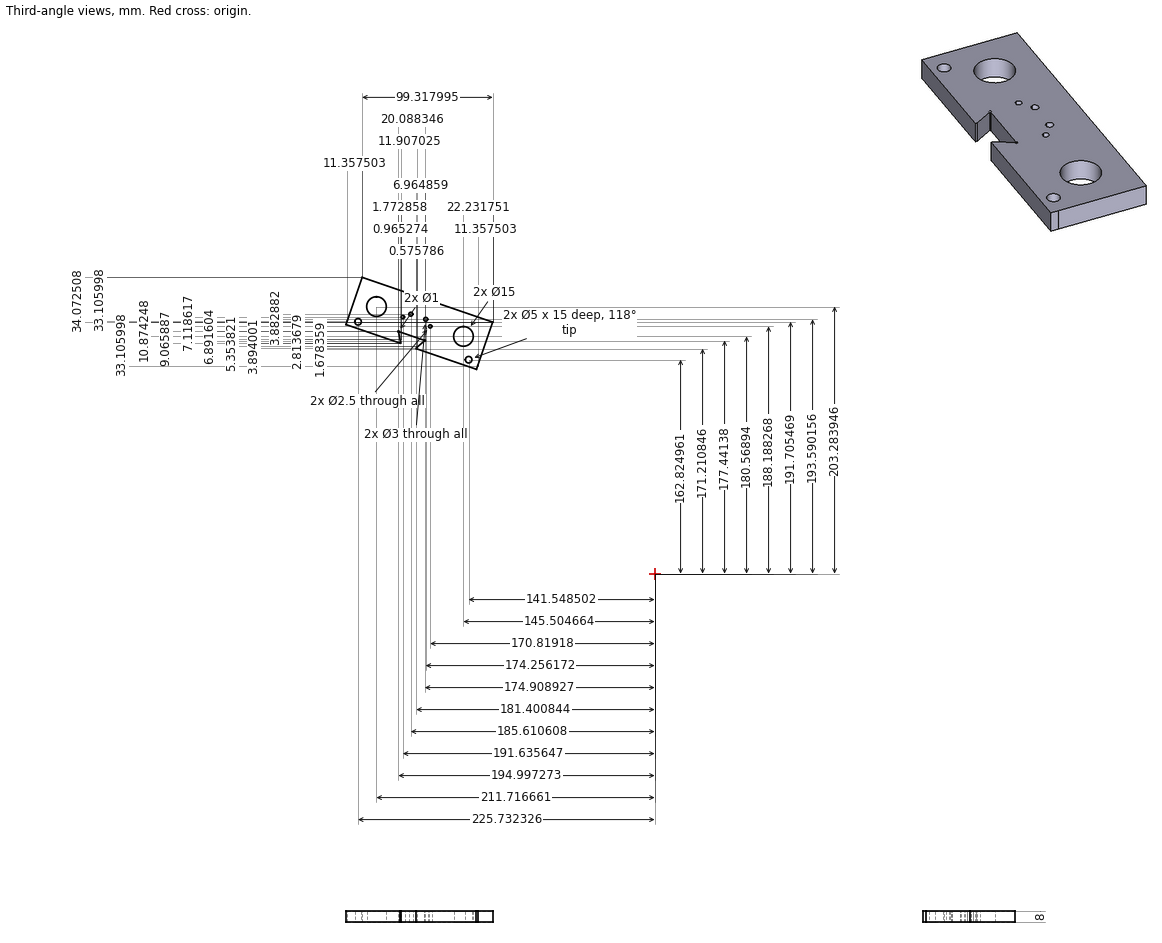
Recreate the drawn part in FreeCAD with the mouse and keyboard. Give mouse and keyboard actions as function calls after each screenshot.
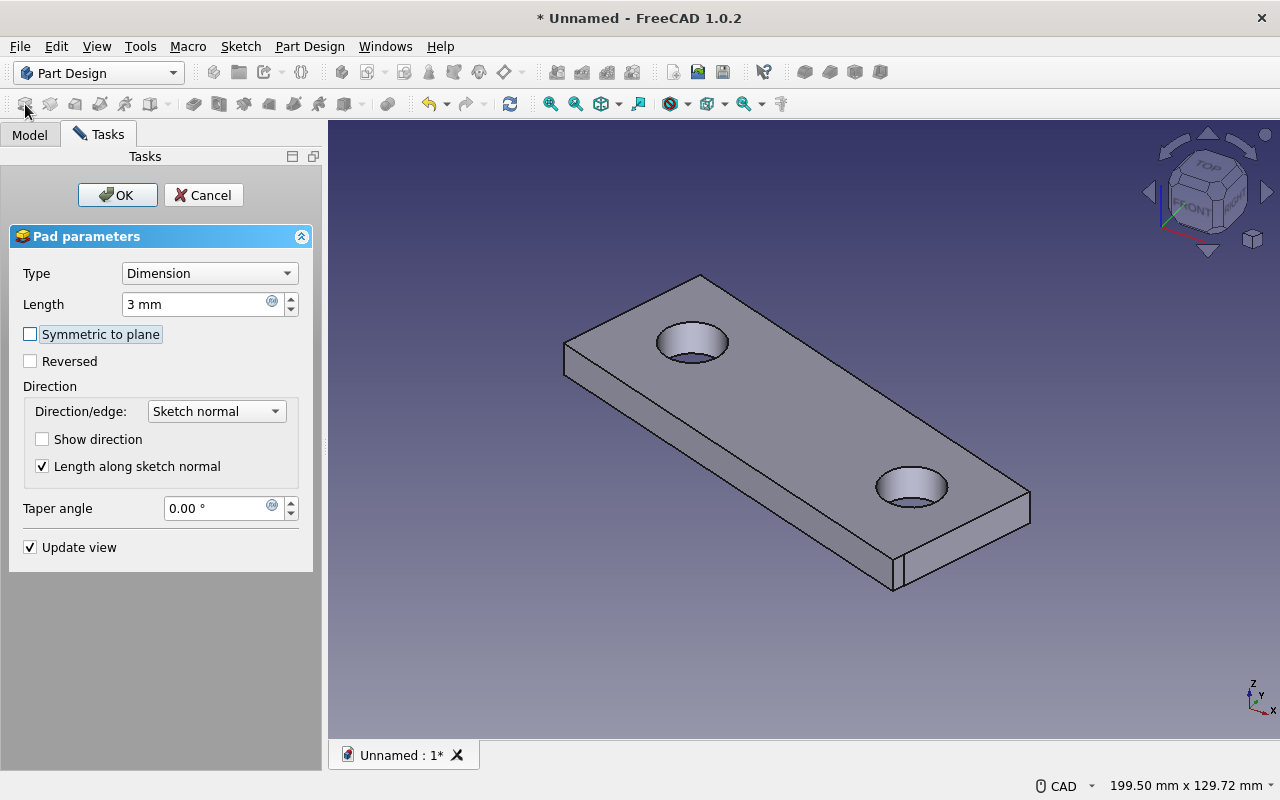
click(118, 195)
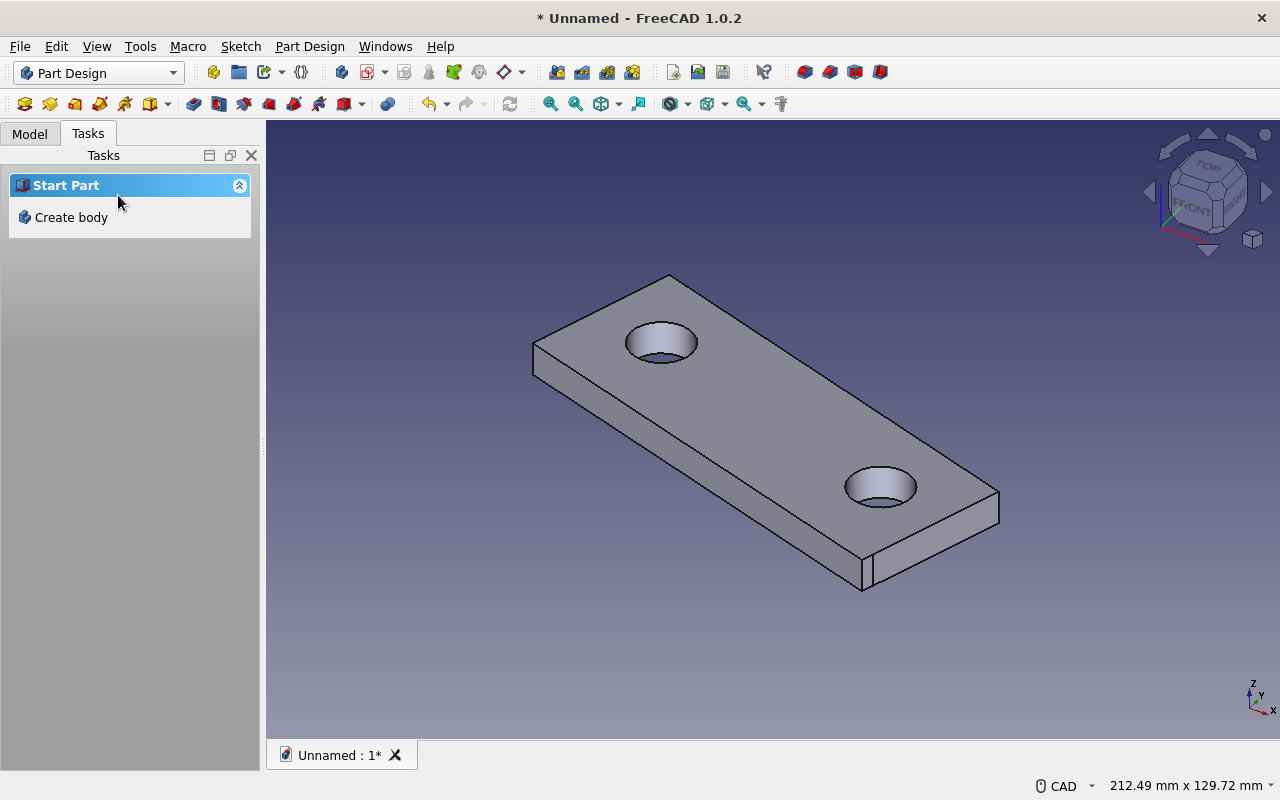
click(766, 416)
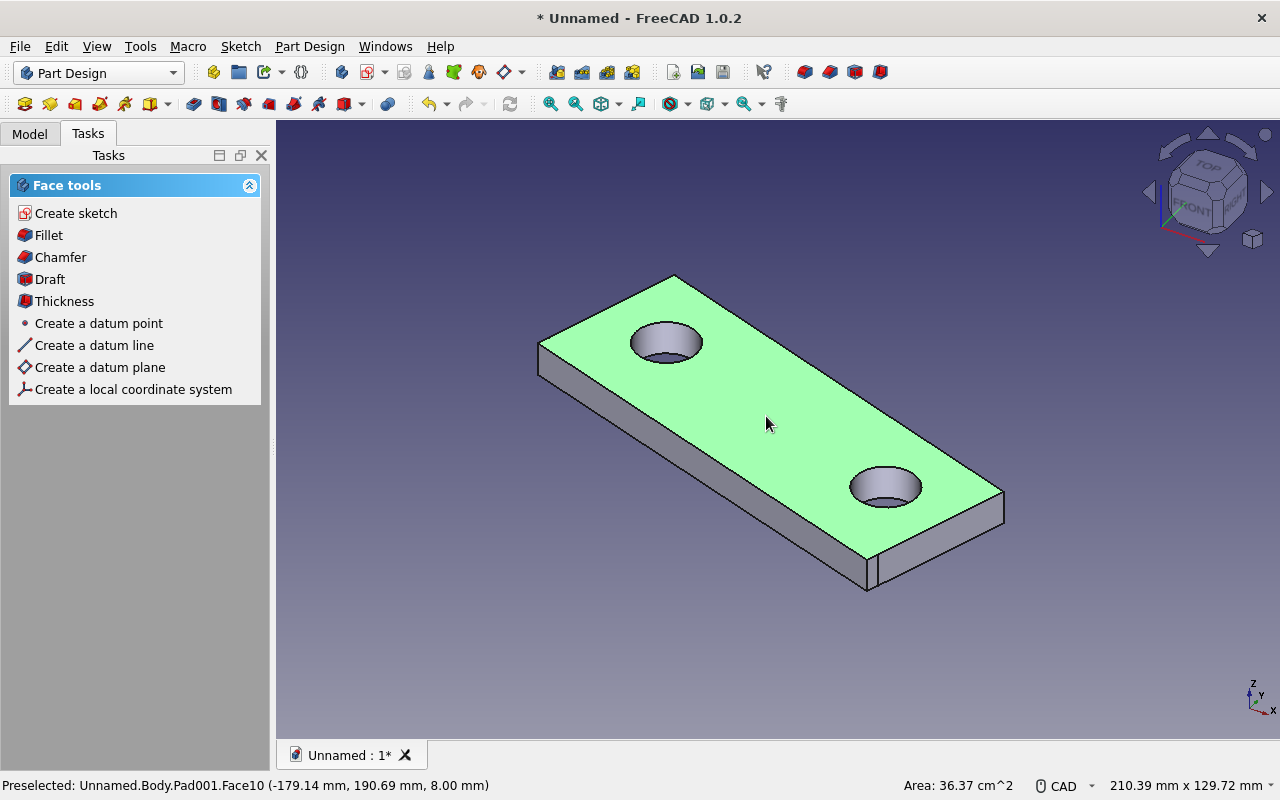
click(366, 72)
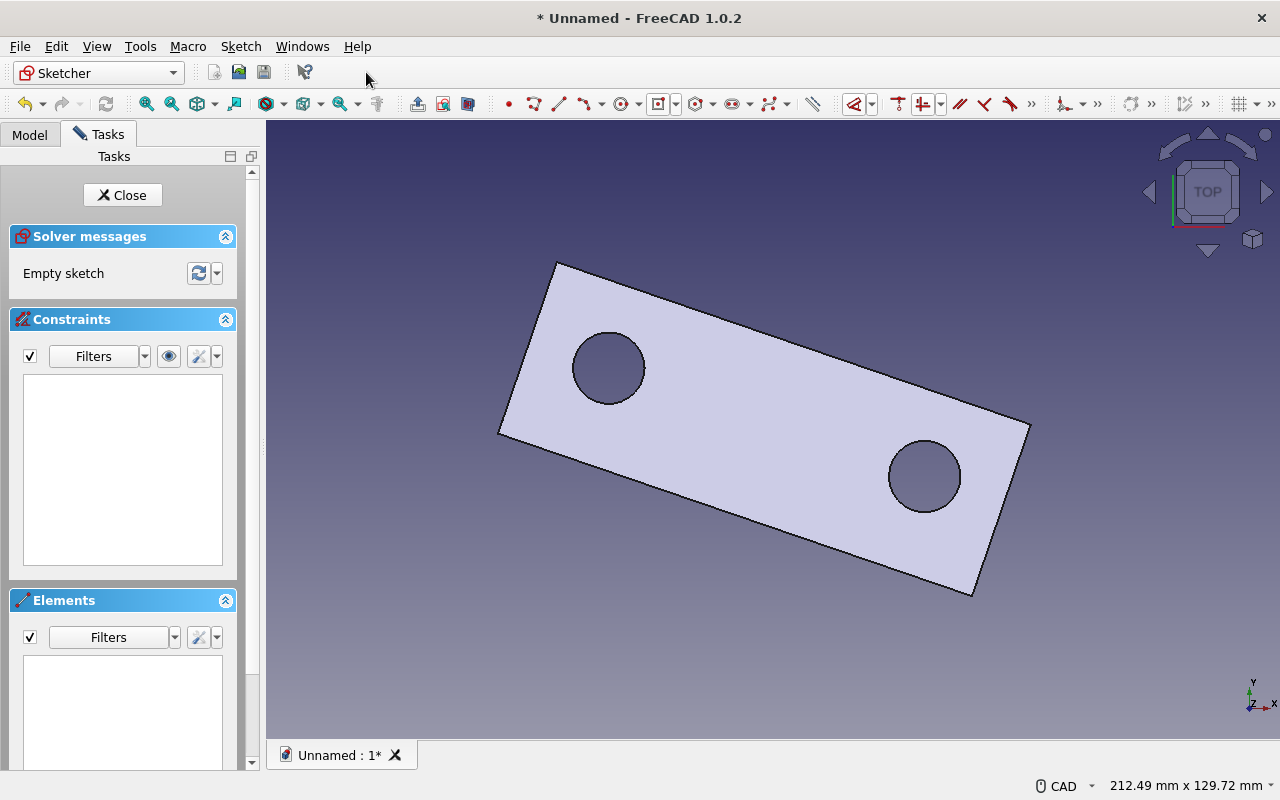
scroll(743, 501, up, 9)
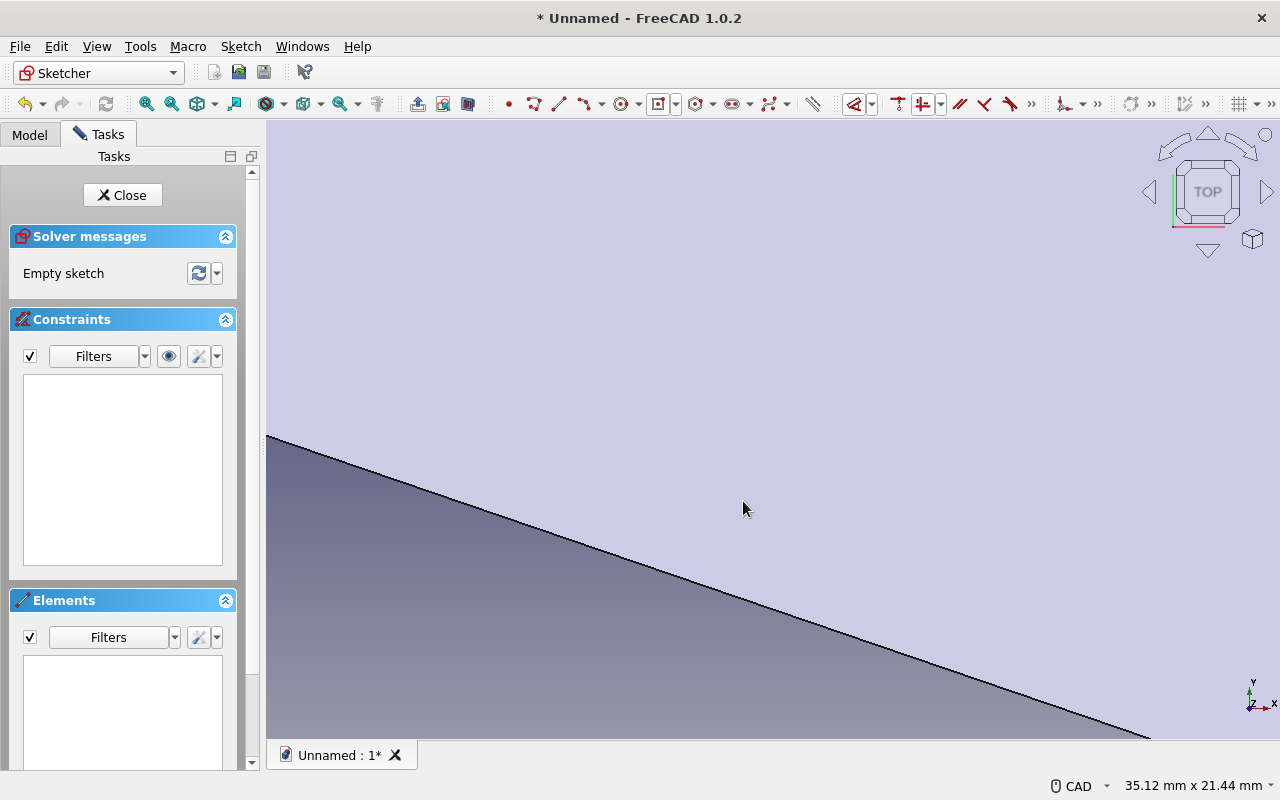
click(534, 104)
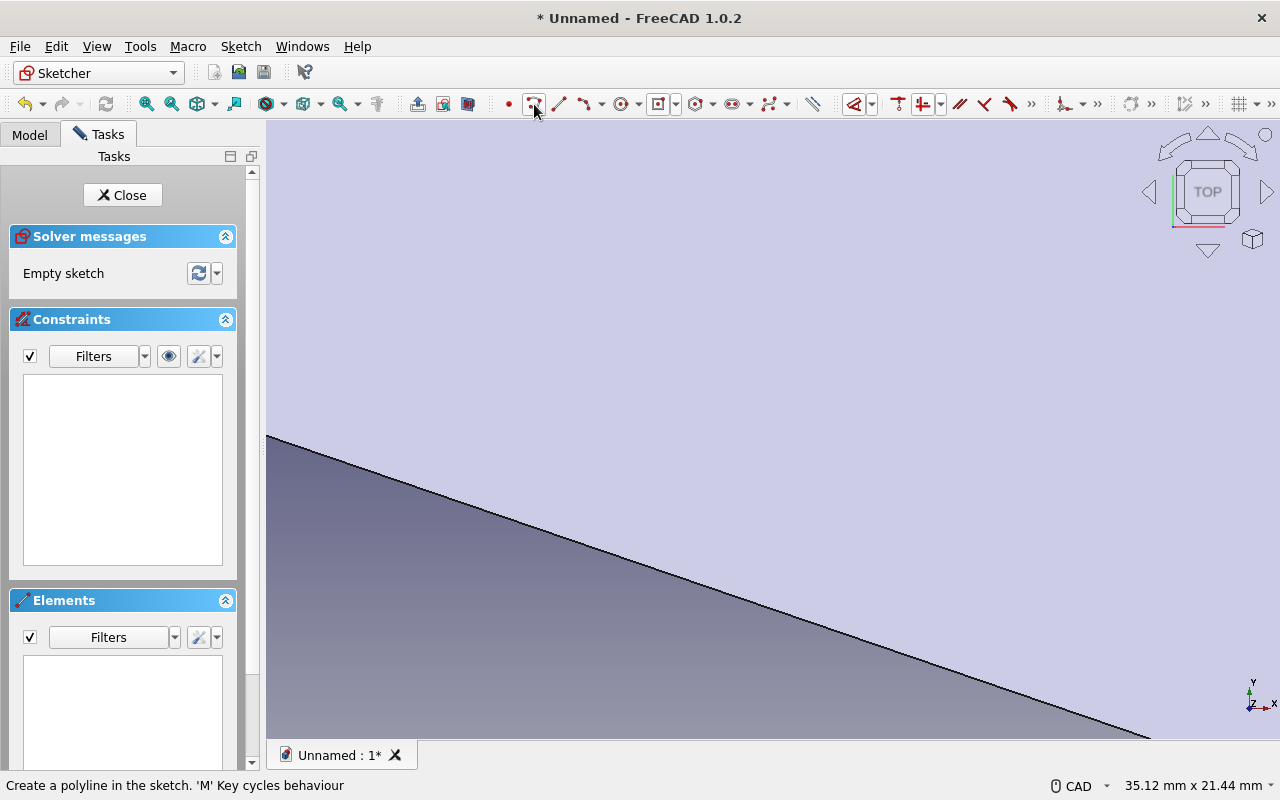
click(991, 440)
click(411, 241)
click(462, 503)
click(790, 615)
click(991, 441)
key(Escape)
key(Escape)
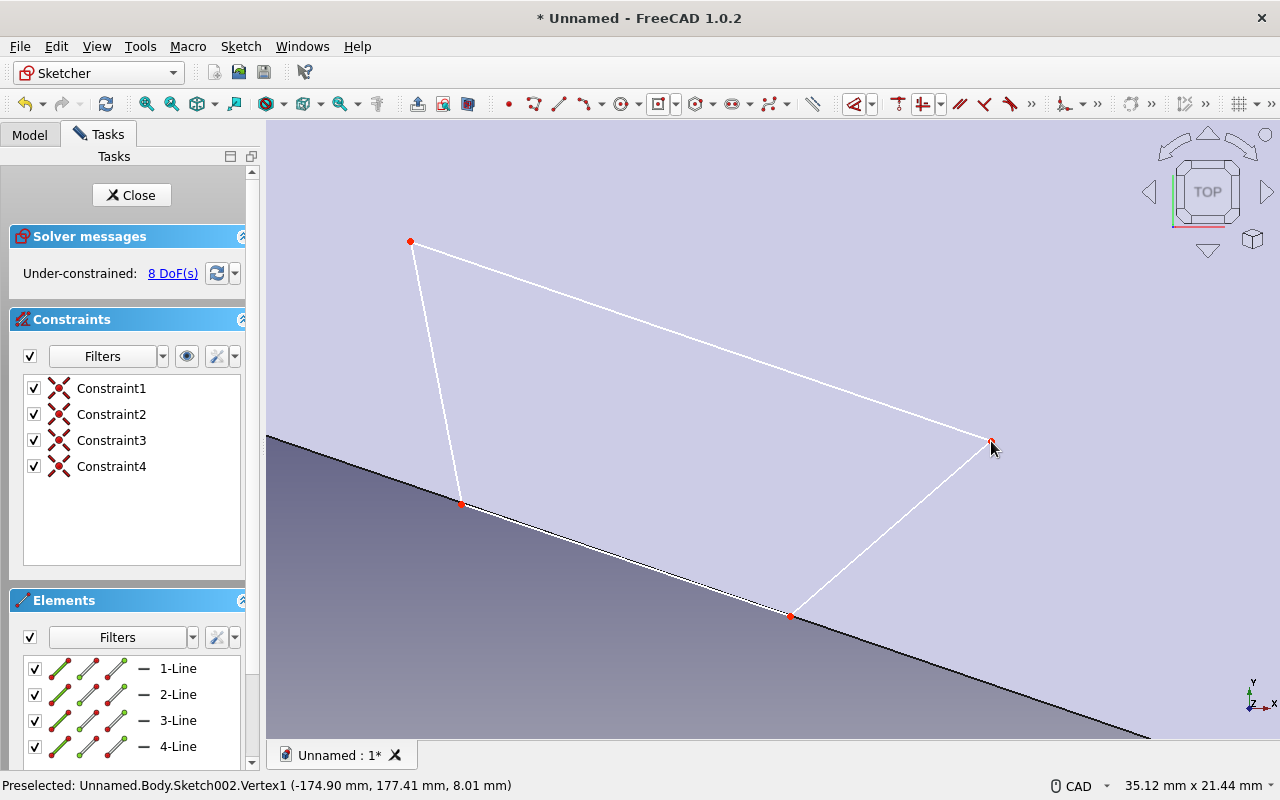
click(817, 381)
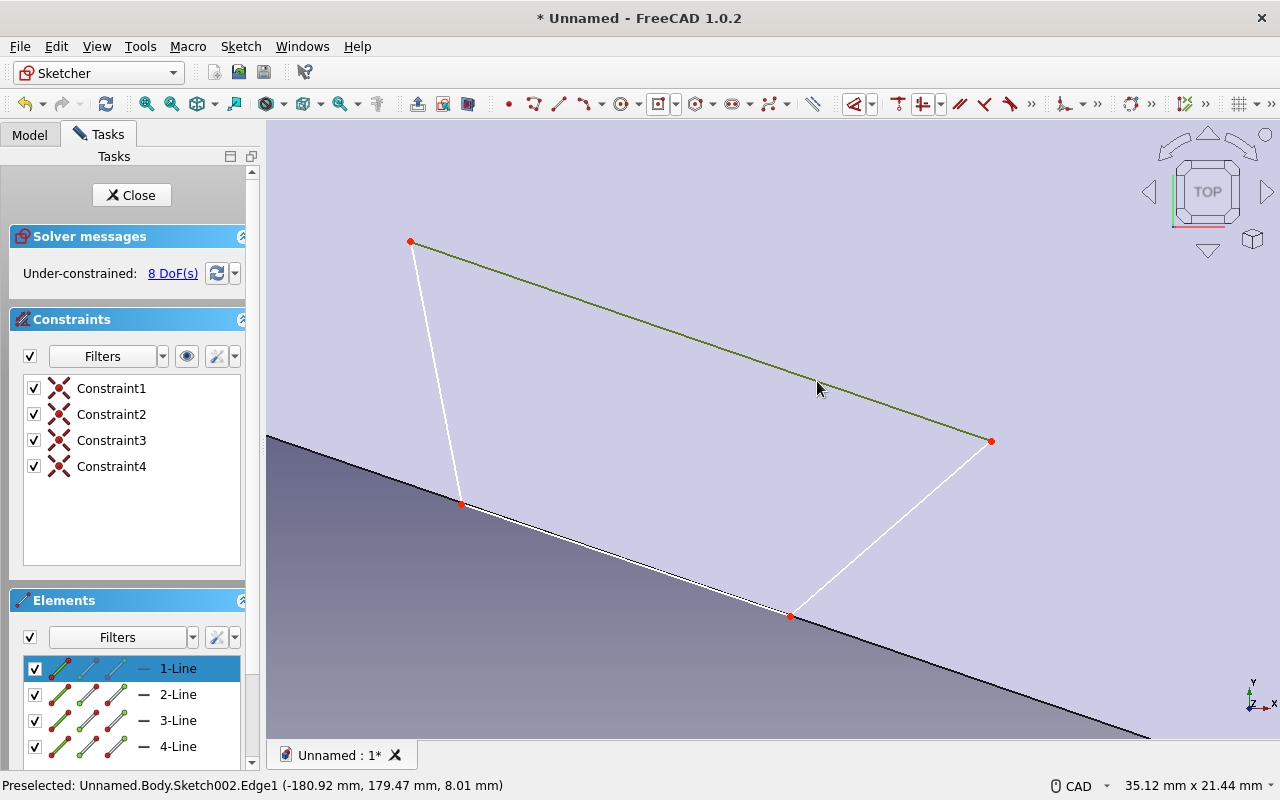
click(872, 104)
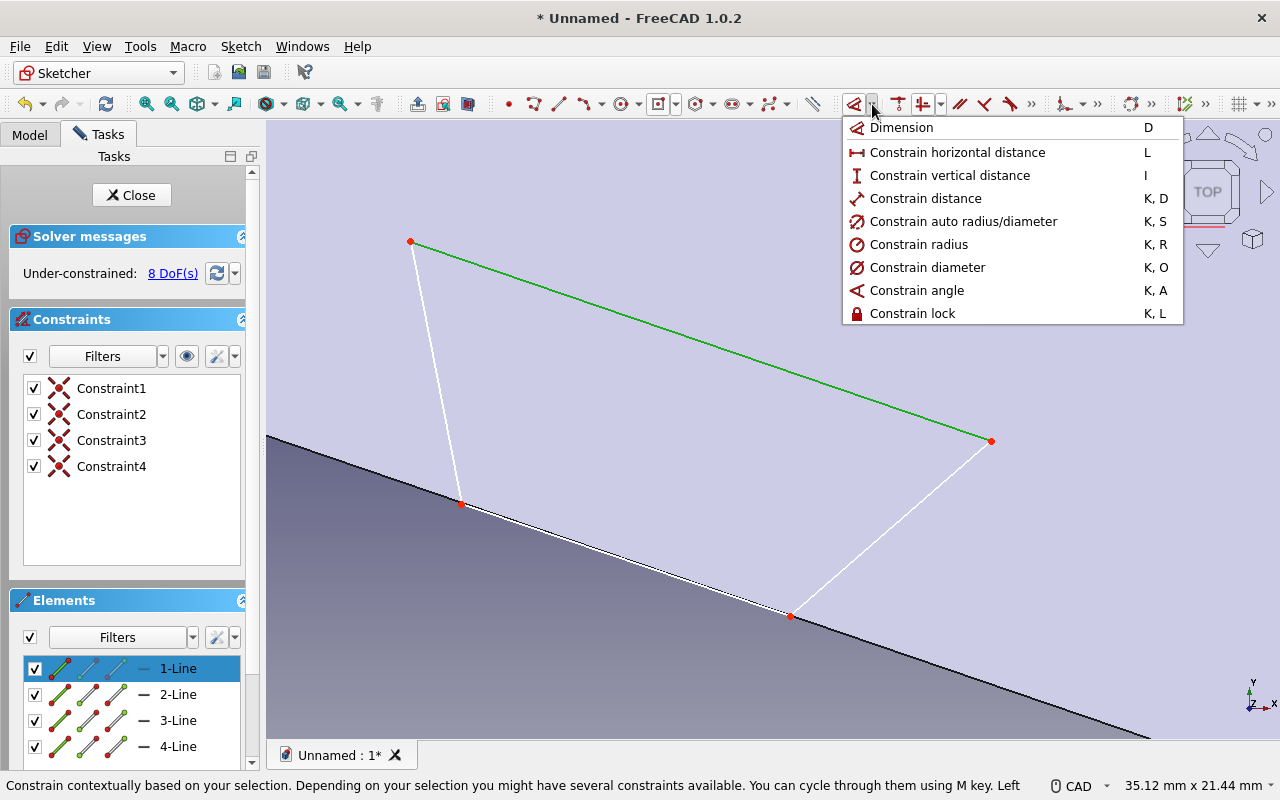
click(1013, 176)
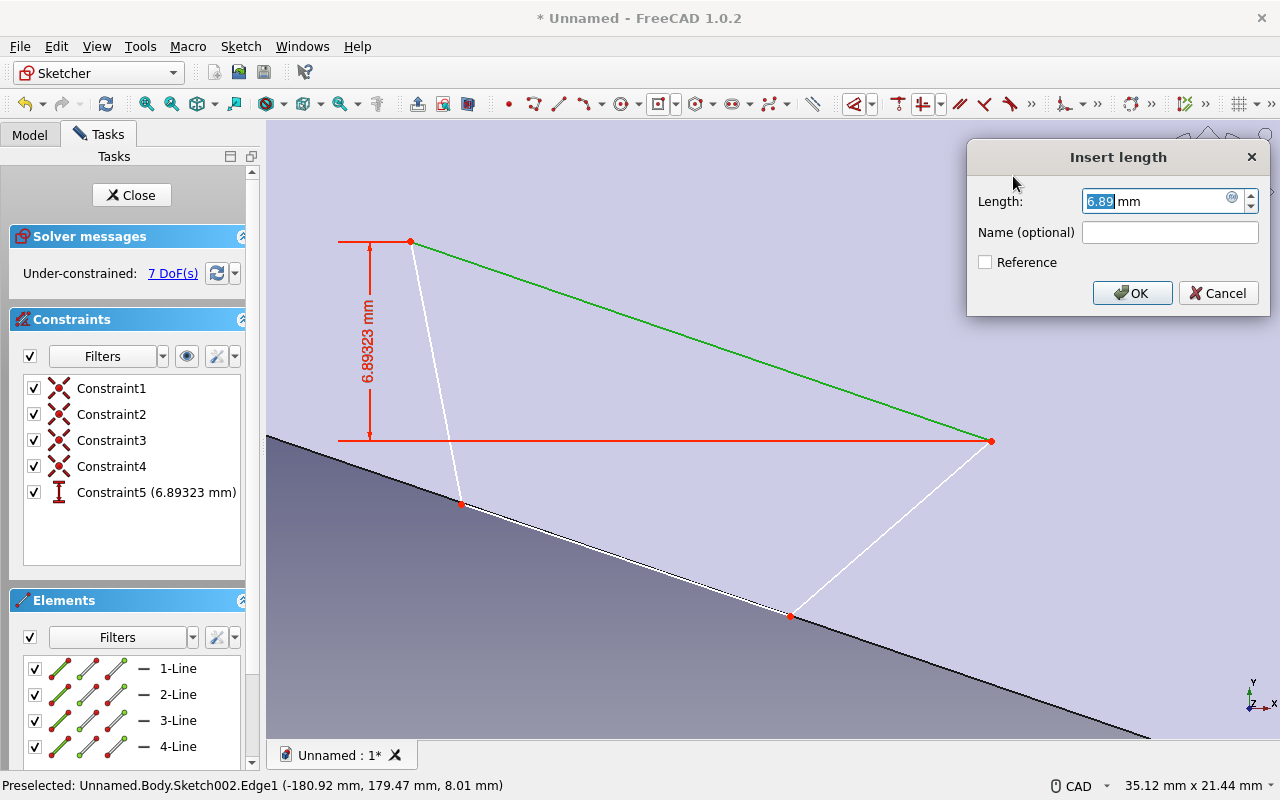
text(6.891604)
key(Return)